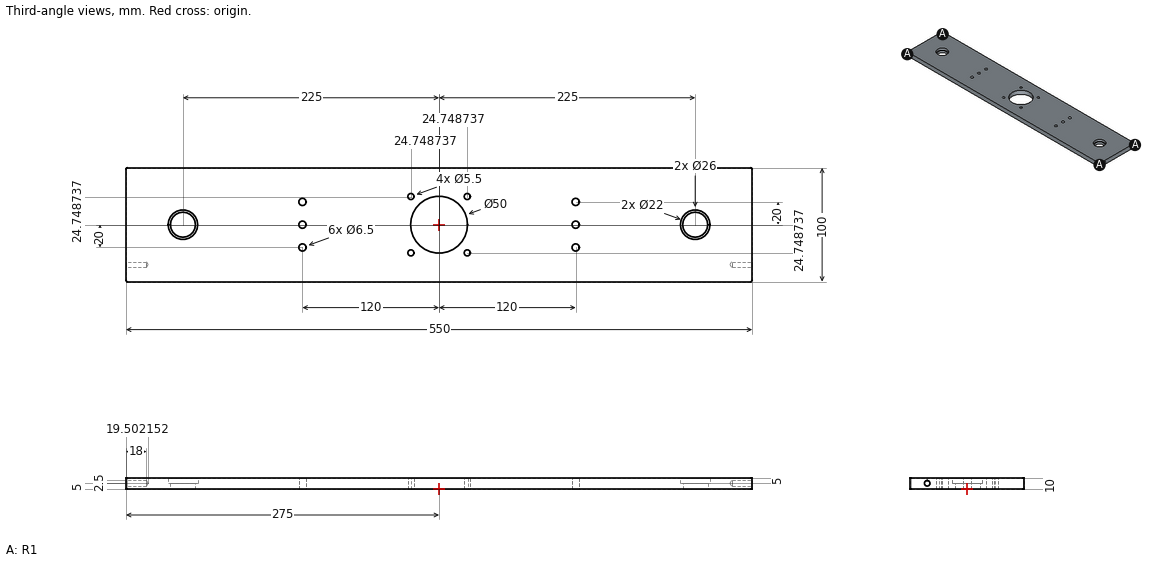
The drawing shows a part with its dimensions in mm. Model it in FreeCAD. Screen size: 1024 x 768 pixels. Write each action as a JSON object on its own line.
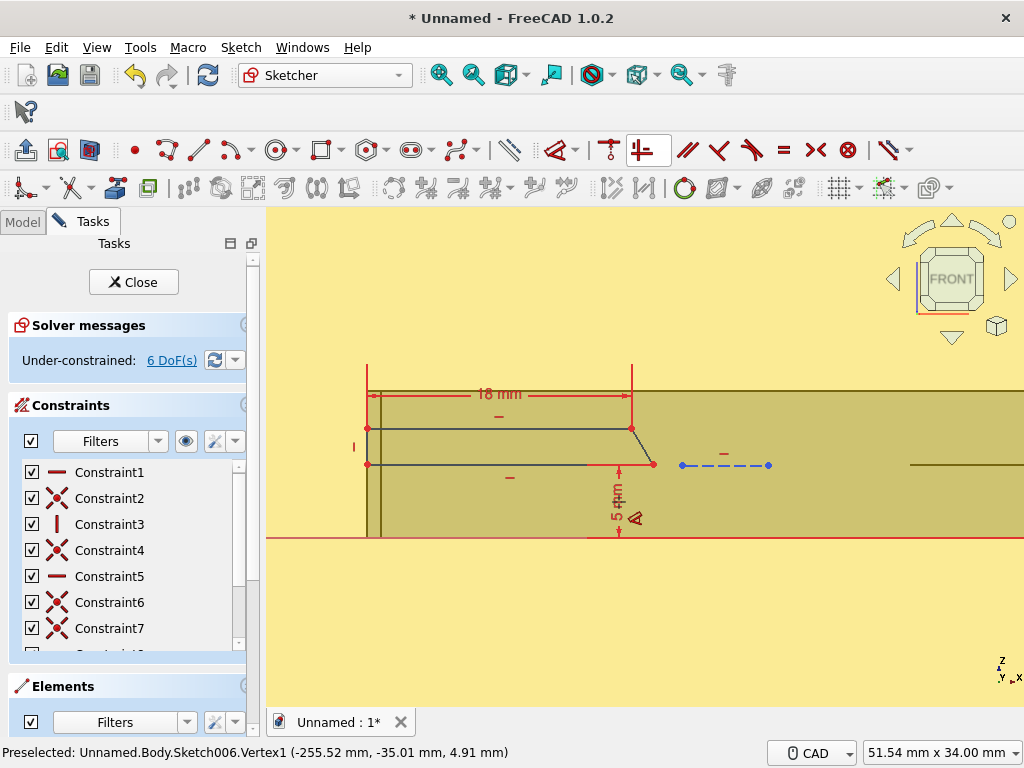
{"action": "left_click", "coordinate": [682, 466]}
{"action": "left_click", "coordinate": [528, 502]}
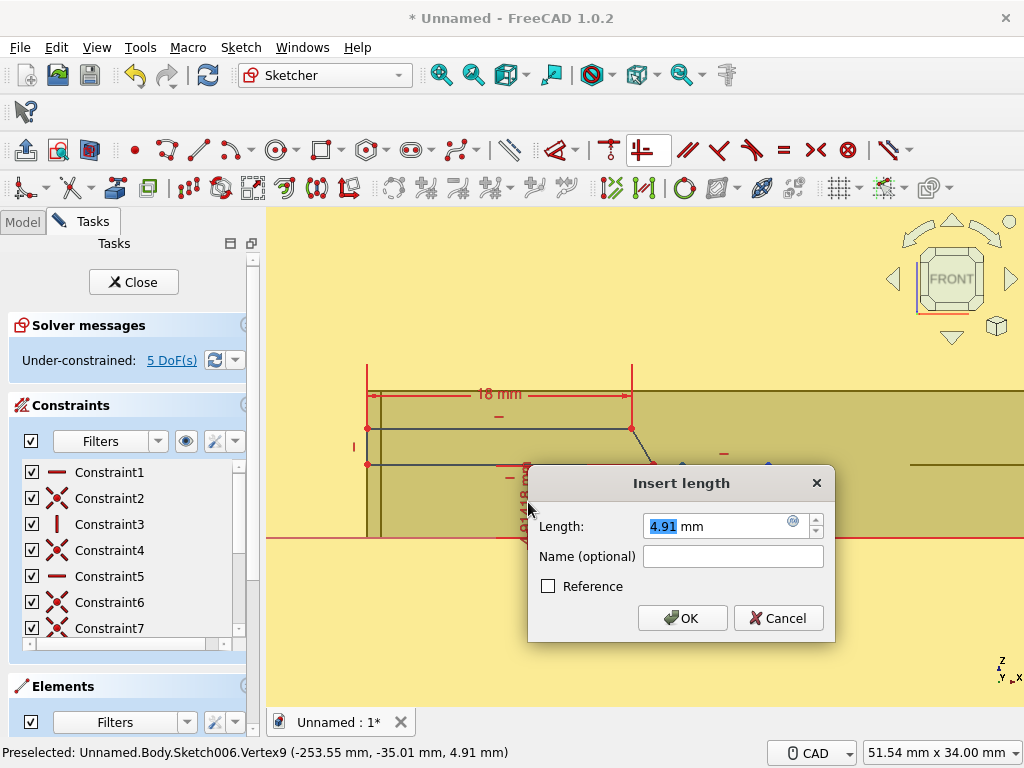
{"action": "type", "text": "5"}
{"action": "key", "text": "Return"}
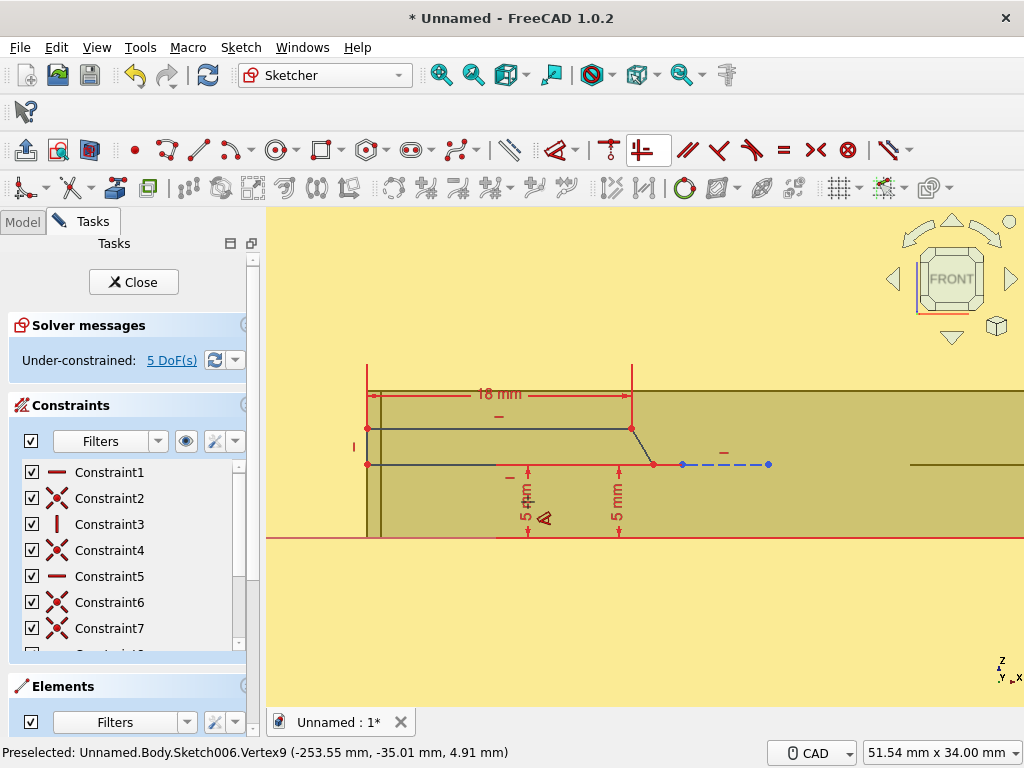
{"action": "scroll", "coordinate": [367, 454], "scroll_direction": "up", "scroll_amount": 2}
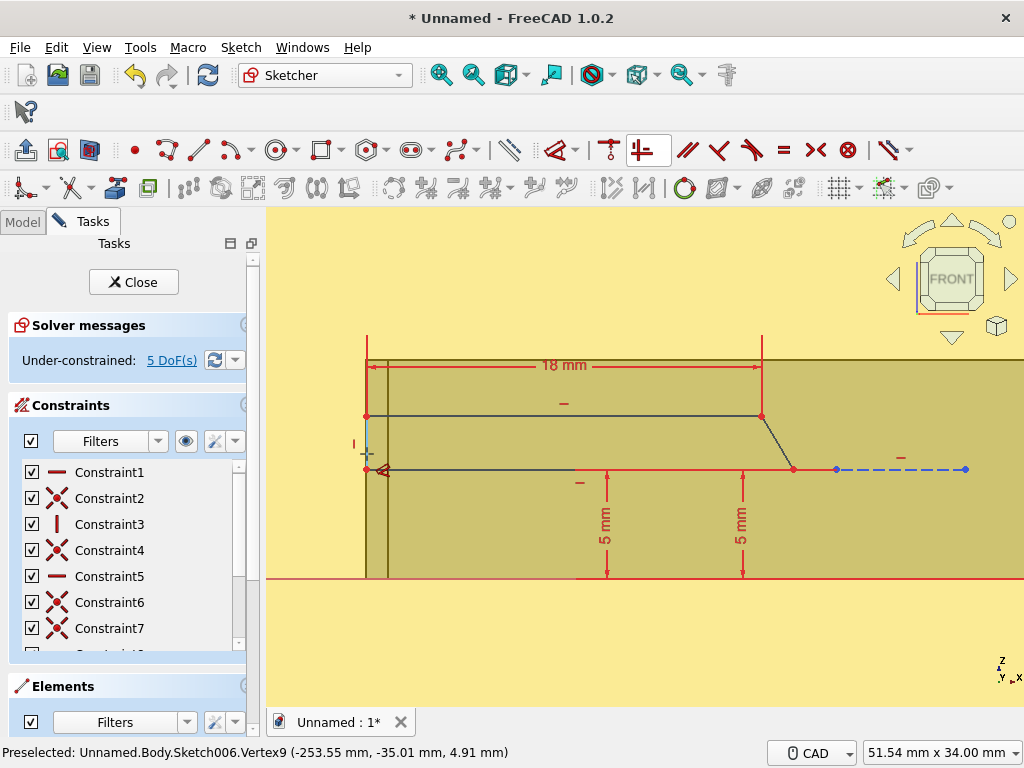
{"action": "left_click", "coordinate": [367, 454]}
{"action": "left_click", "coordinate": [333, 443]}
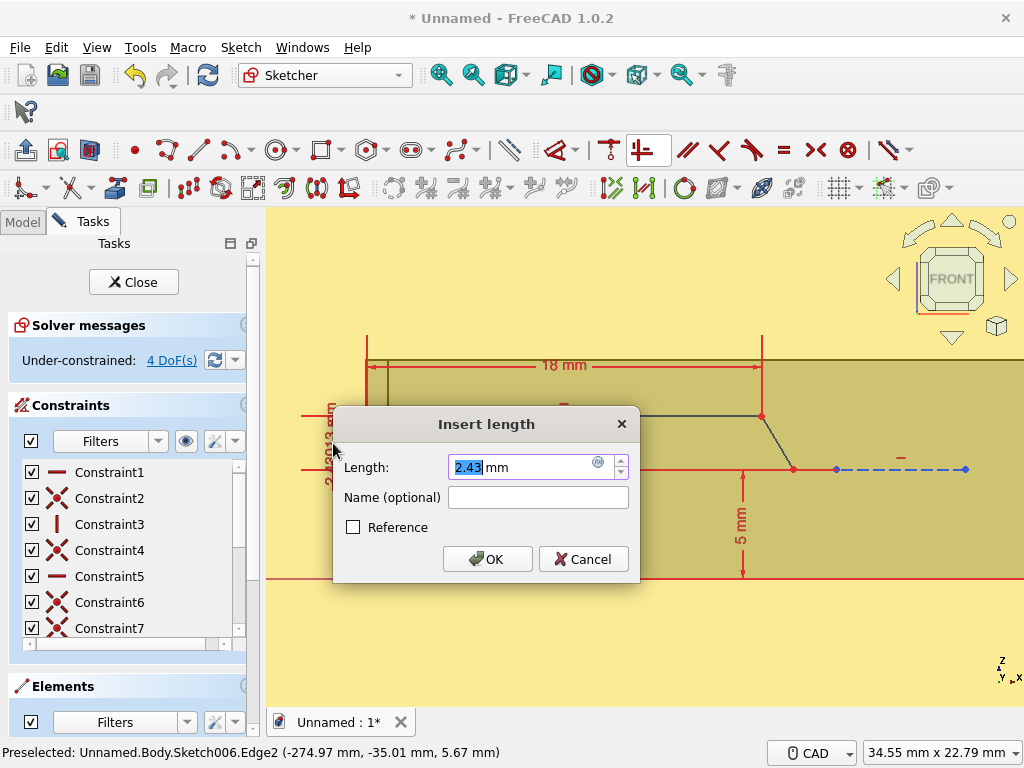
{"action": "type", "text": "2.5"}
{"action": "key", "text": "Return"}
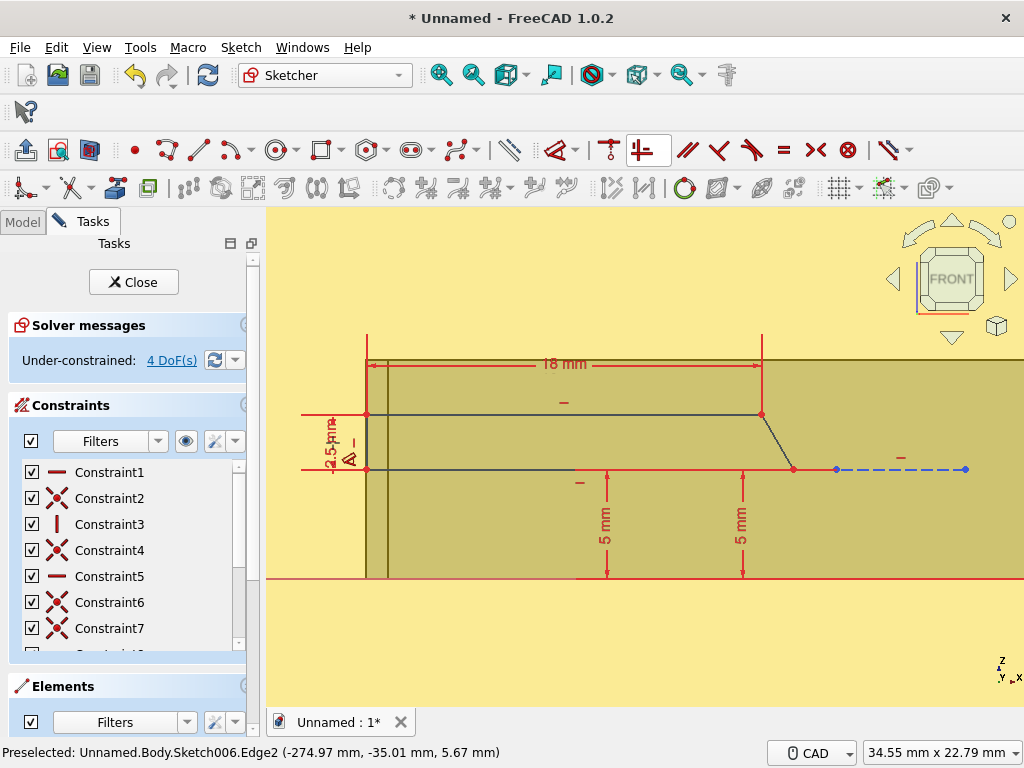
{"action": "left_click", "coordinate": [367, 470]}
{"action": "left_click", "coordinate": [613, 613]}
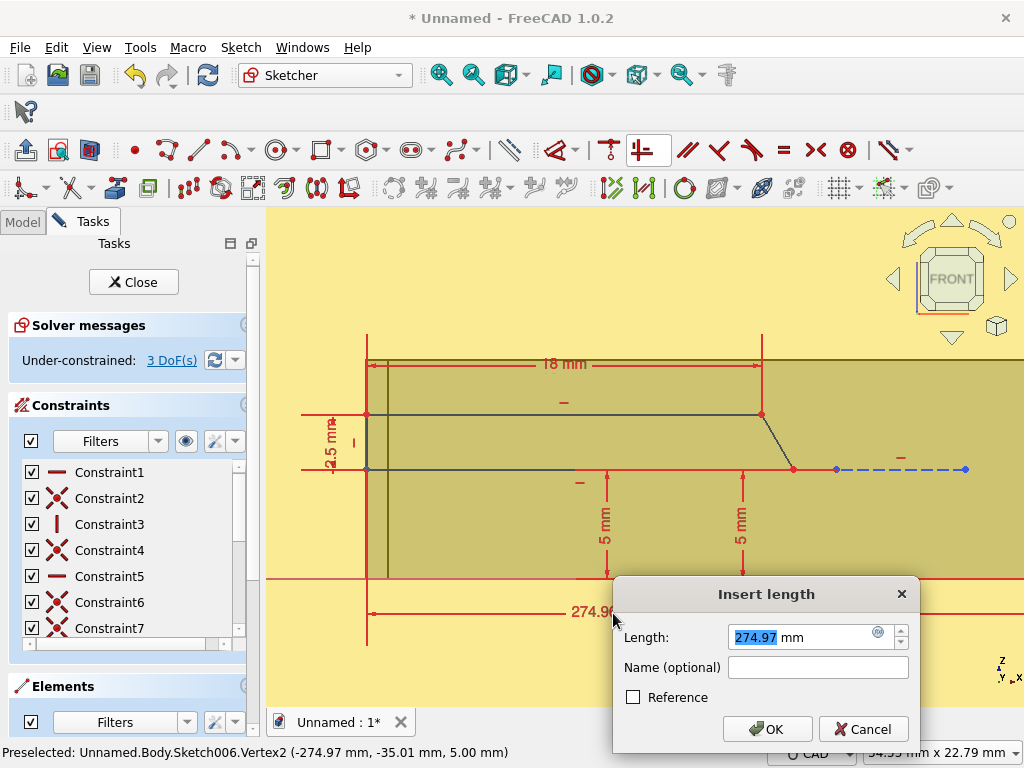
{"action": "type", "text": "275"}
{"action": "key", "text": "Return"}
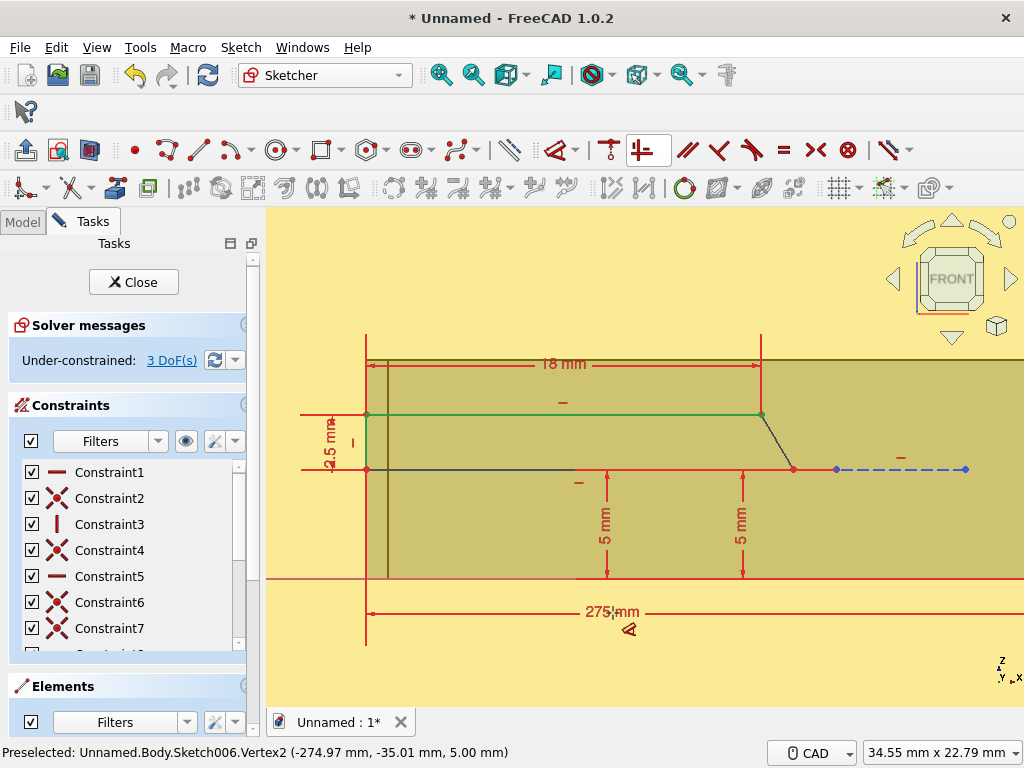
{"action": "left_click", "coordinate": [665, 470]}
{"action": "left_click", "coordinate": [580, 504]}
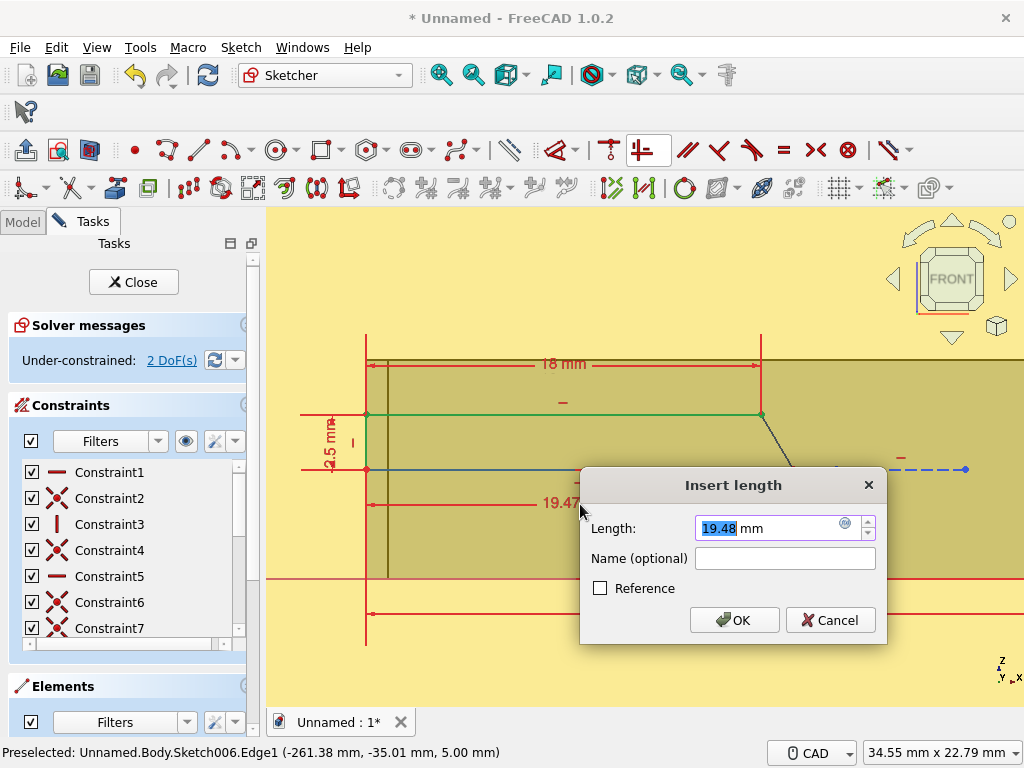
{"action": "type", "text": "19.502152"}
{"action": "key", "text": "Return"}
{"action": "key", "text": "Escape"}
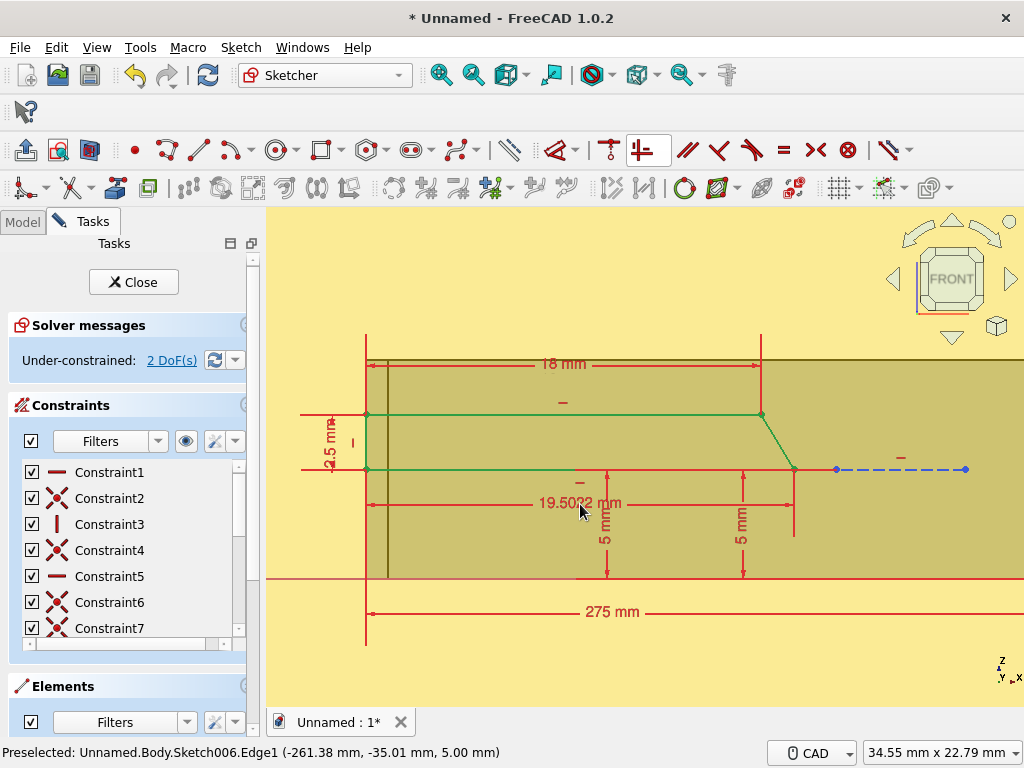
{"action": "left_click", "coordinate": [134, 282]}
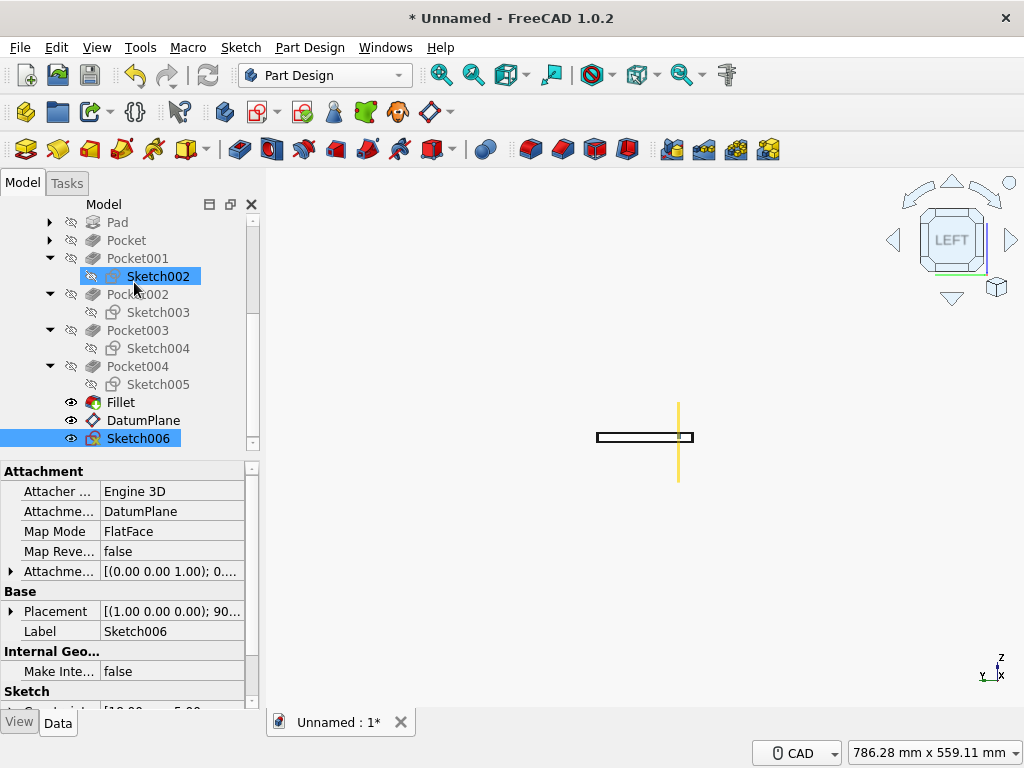
{"action": "left_click", "coordinate": [304, 150]}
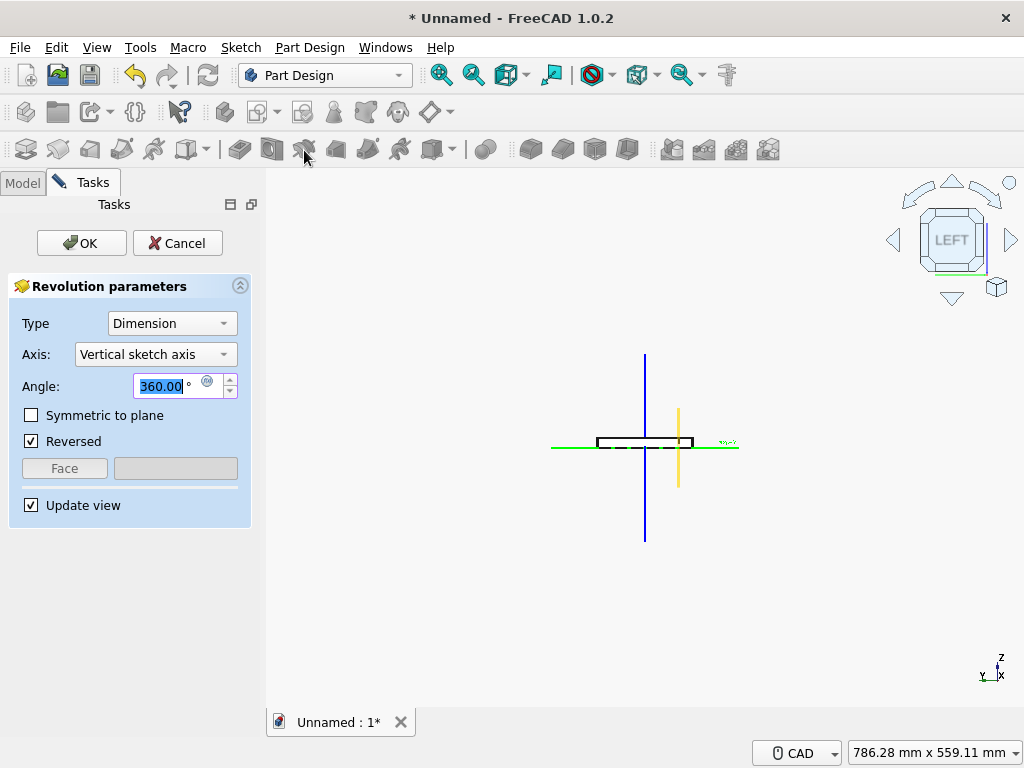
{"action": "left_click", "coordinate": [156, 354]}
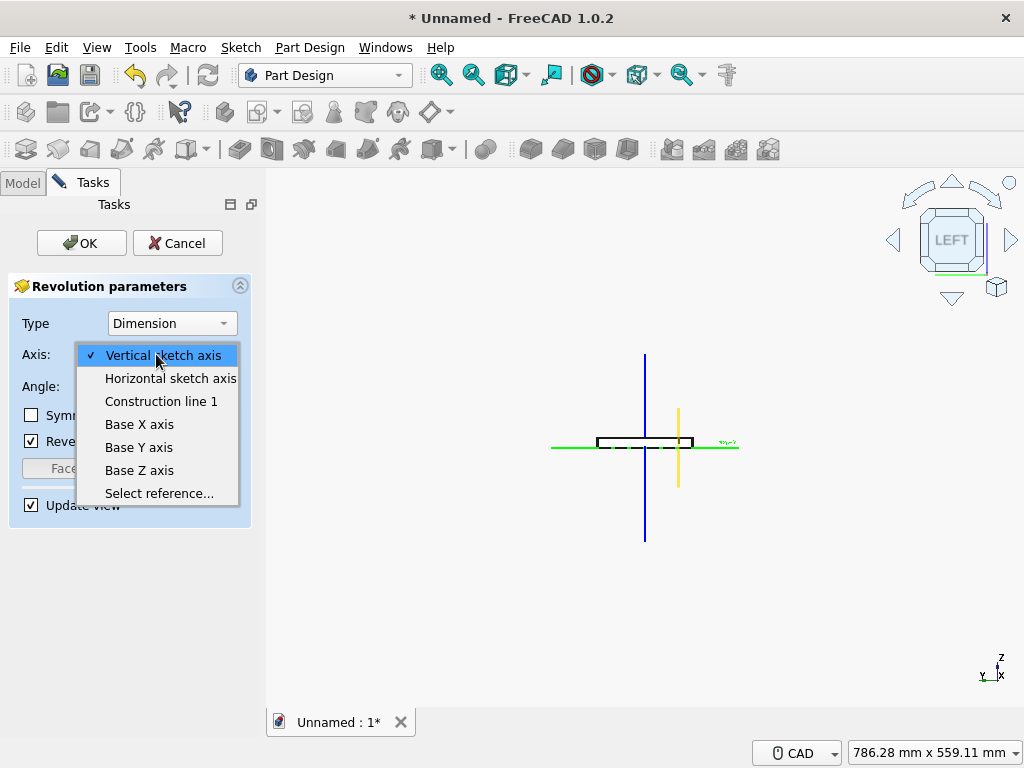
{"action": "left_click", "coordinate": [156, 402]}